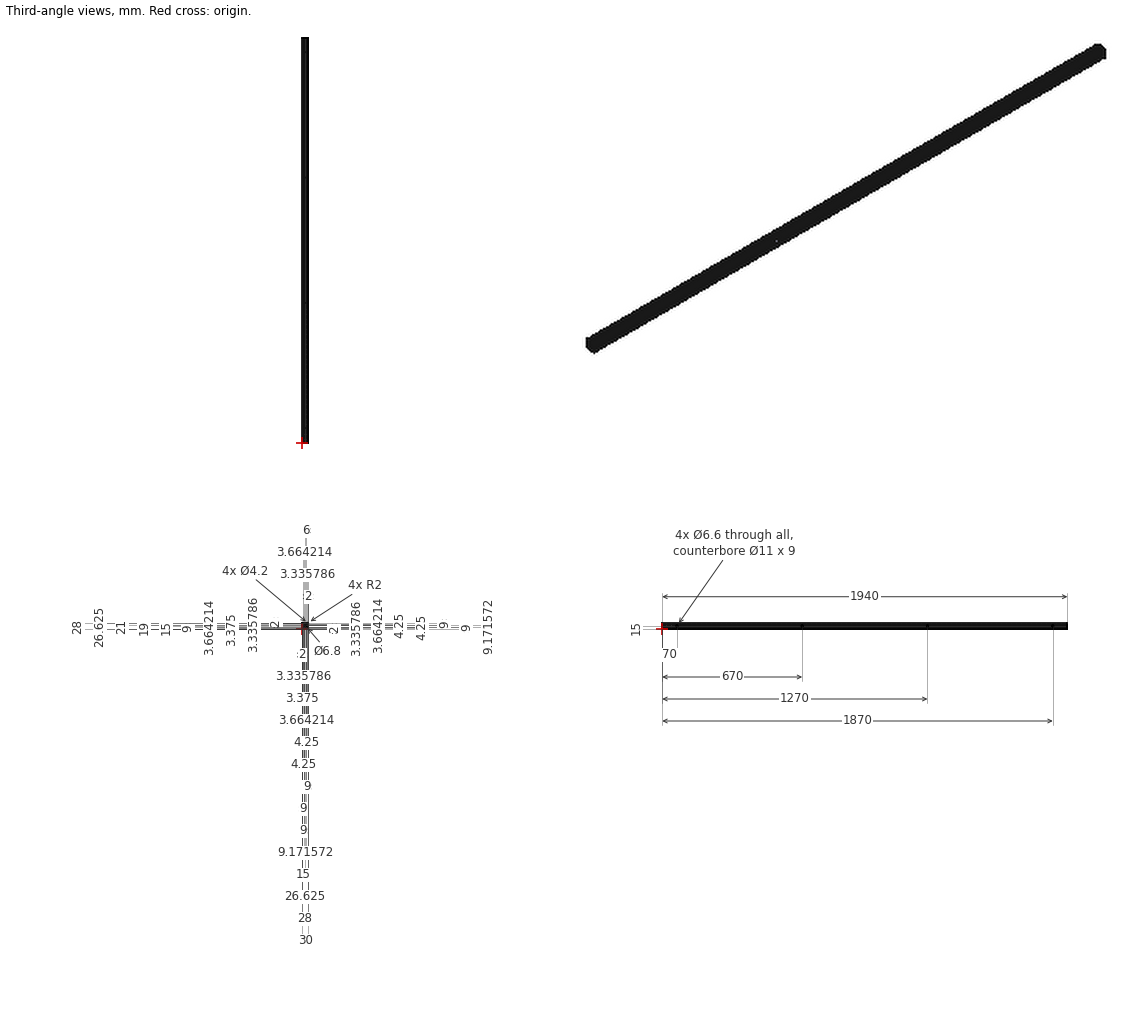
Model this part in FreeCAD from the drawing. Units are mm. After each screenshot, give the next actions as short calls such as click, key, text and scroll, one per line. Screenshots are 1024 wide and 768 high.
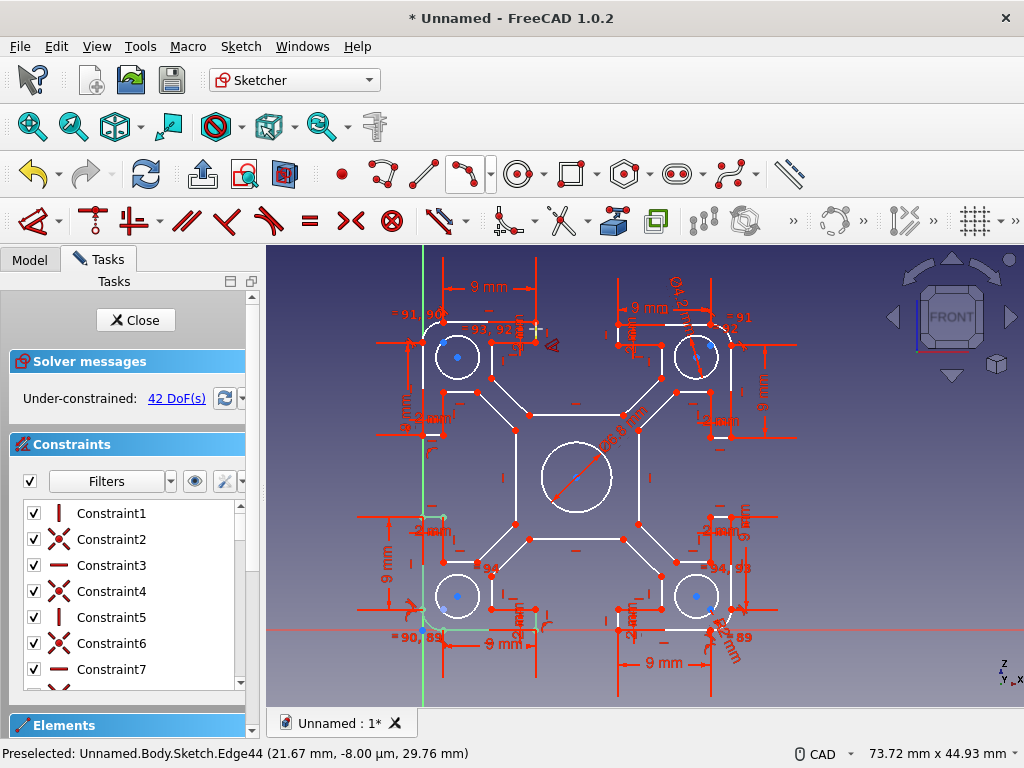
click(624, 539)
click(389, 585)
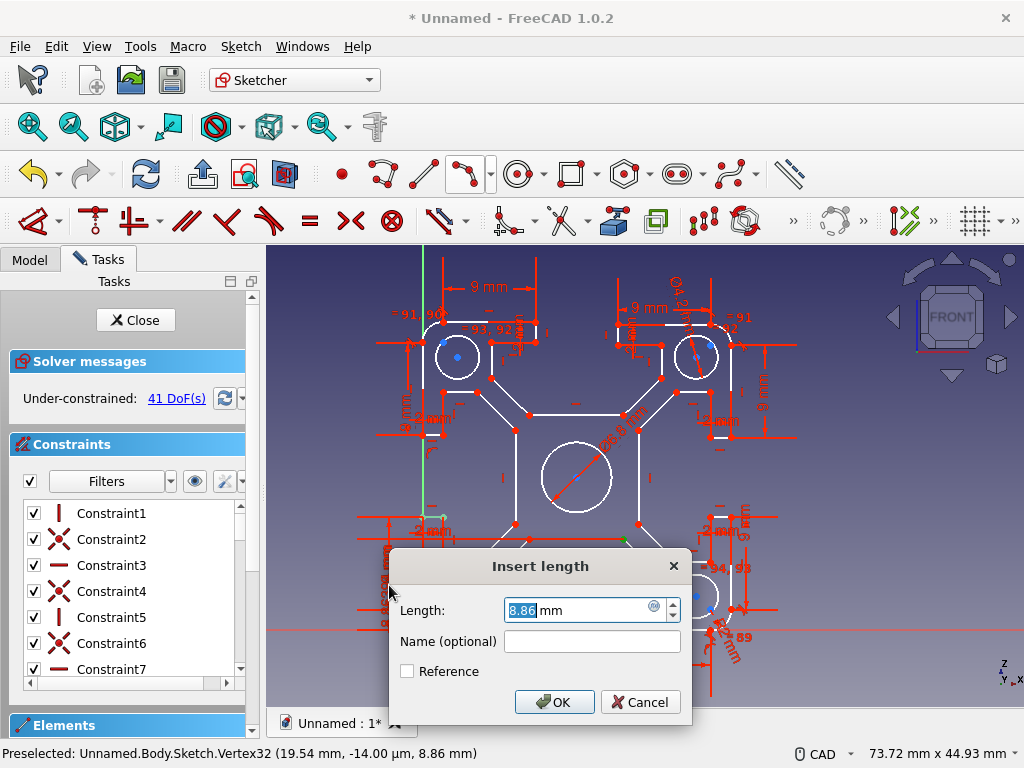
text(9)
key(Return)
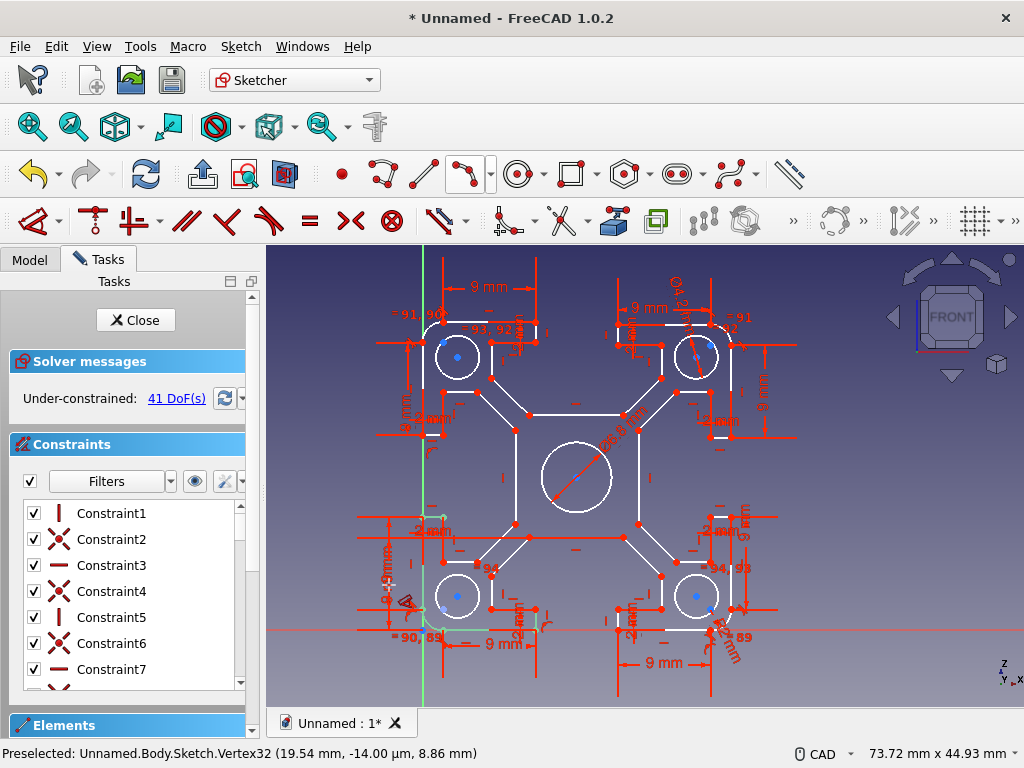
click(516, 524)
click(469, 490)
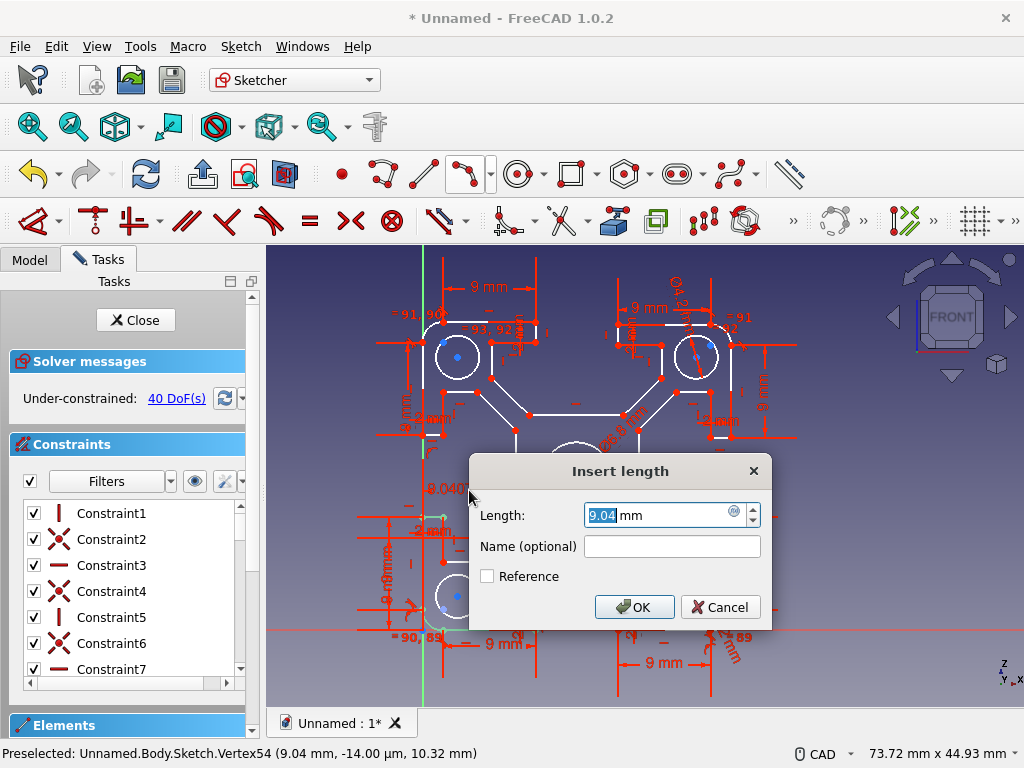
text(9)
key(Return)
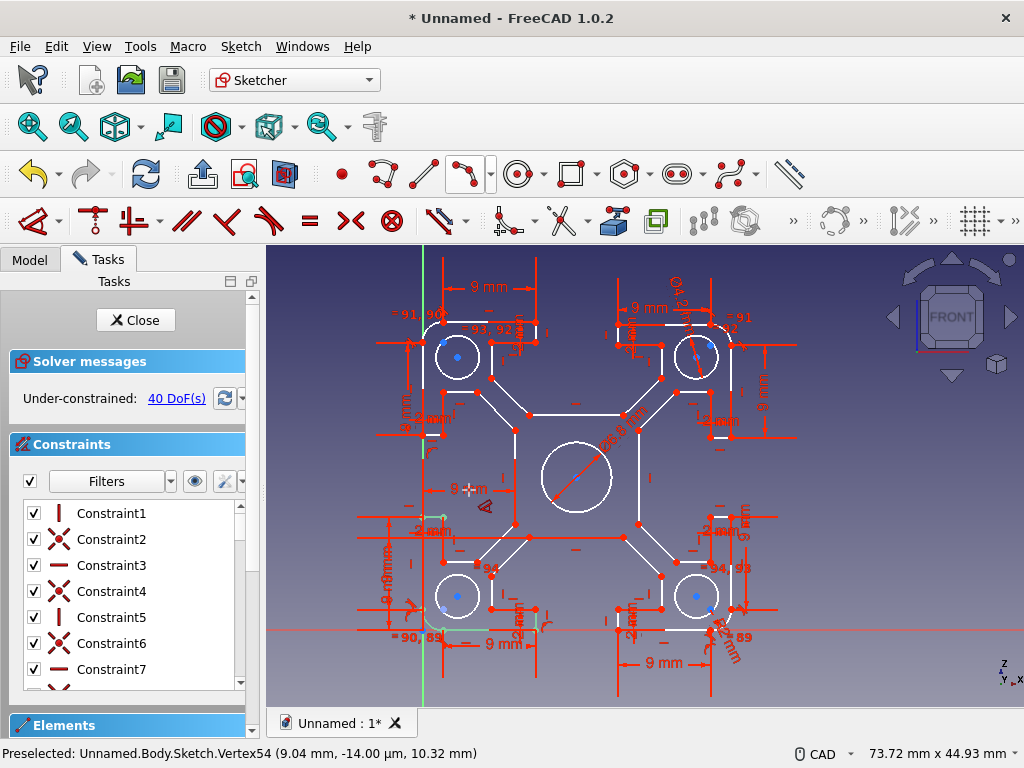
click(577, 477)
click(500, 443)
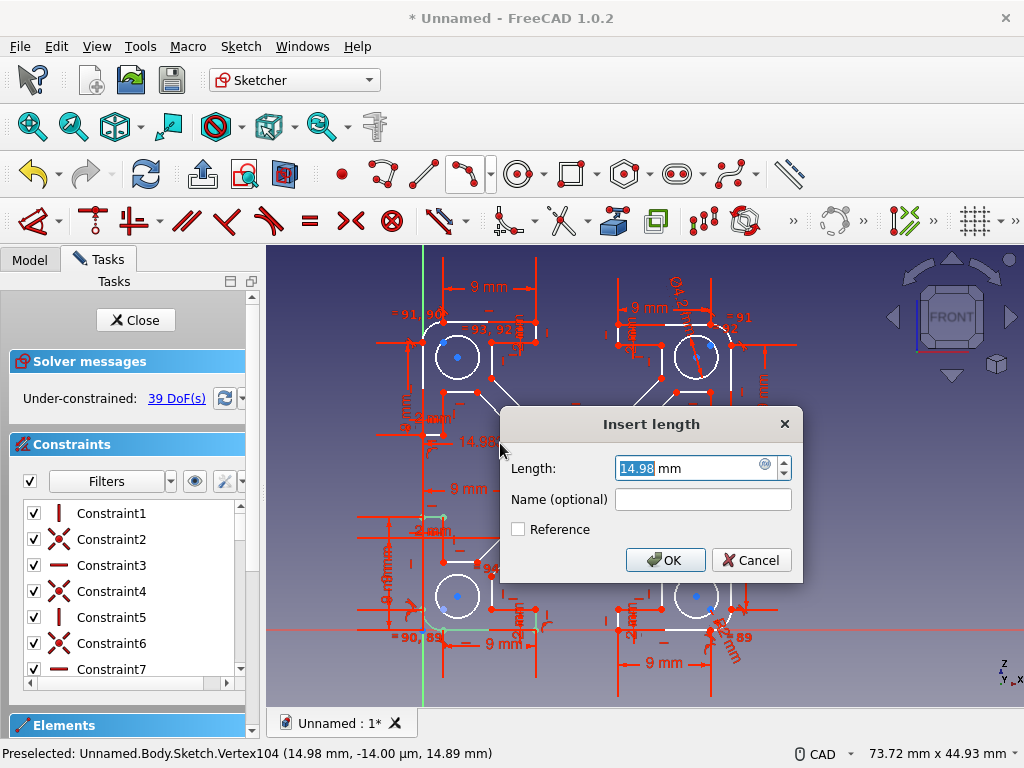
text(15)
key(Return)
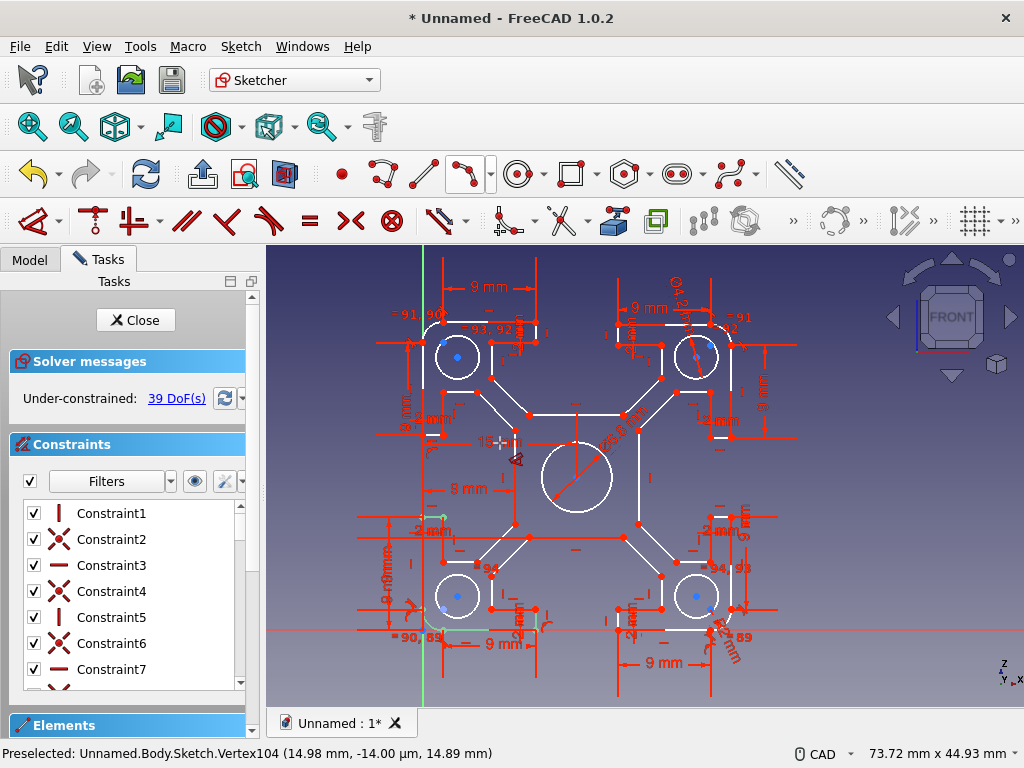
click(577, 477)
click(389, 500)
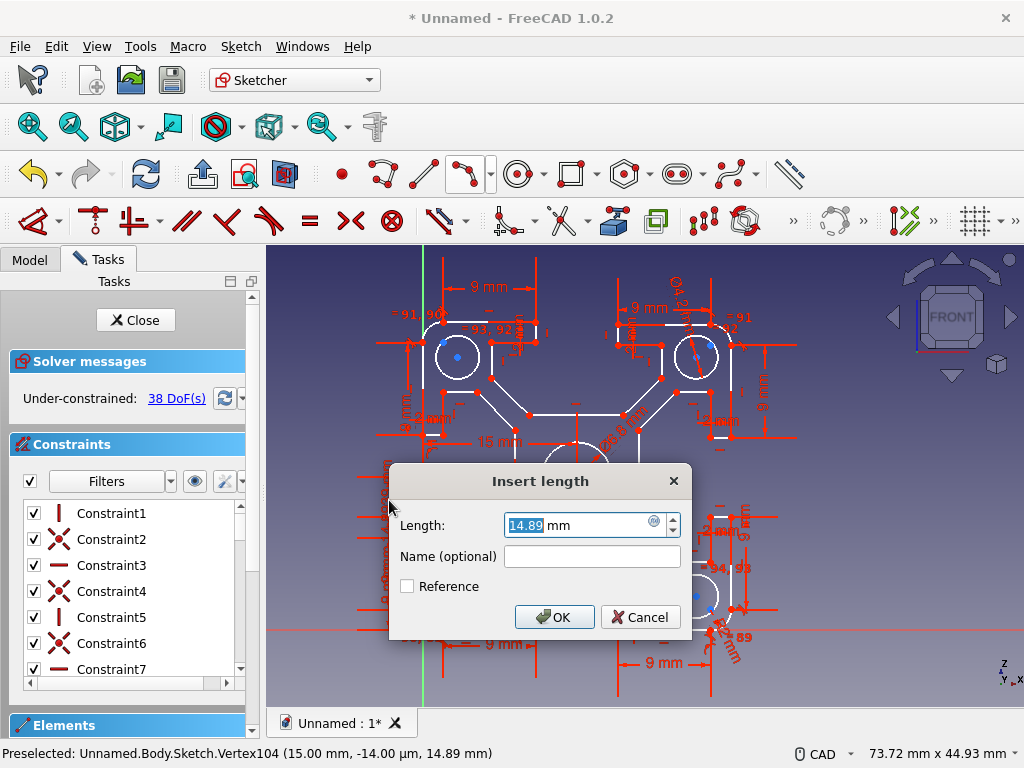
text(15)
key(Return)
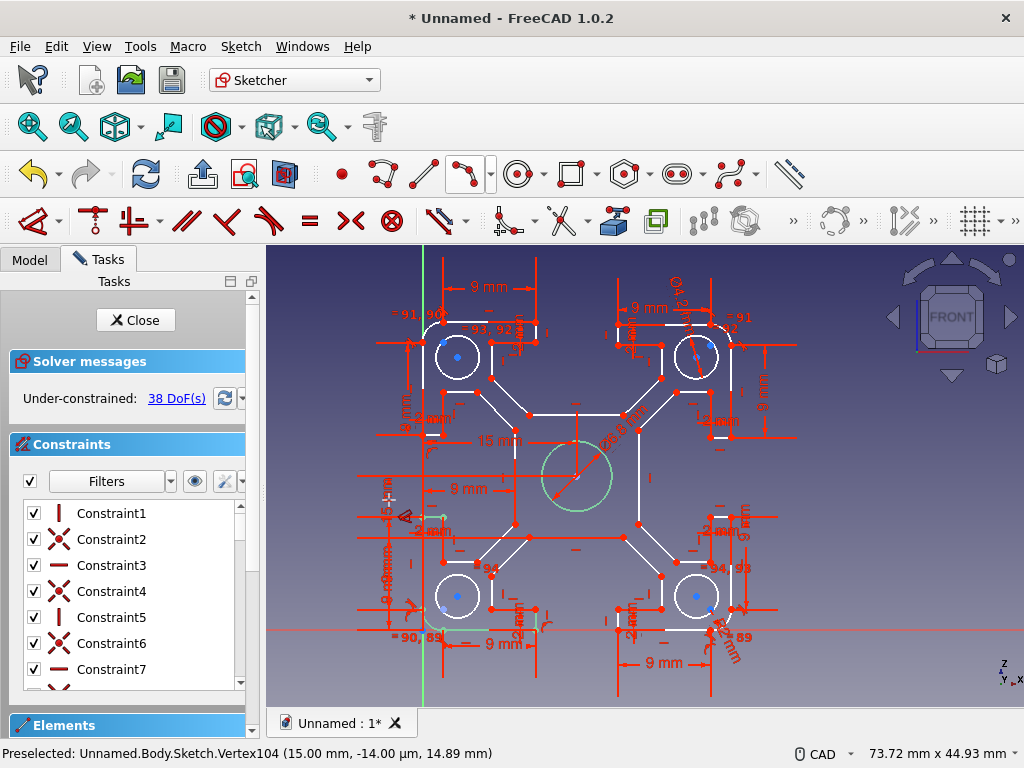
click(639, 430)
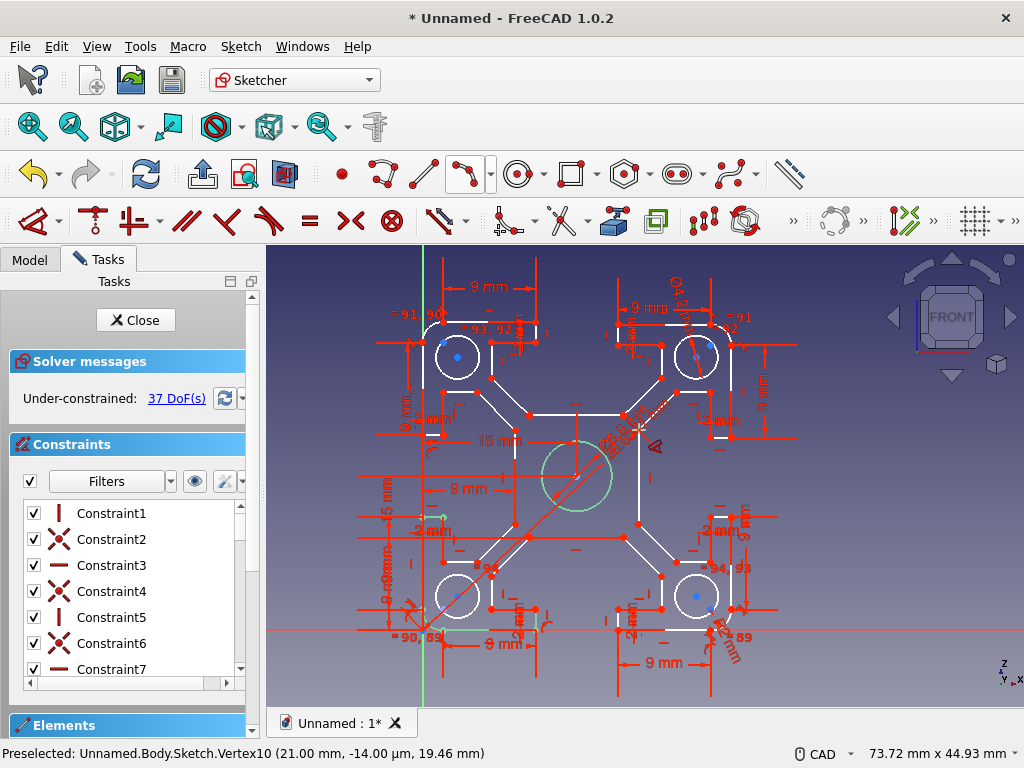
click(577, 476)
click(608, 396)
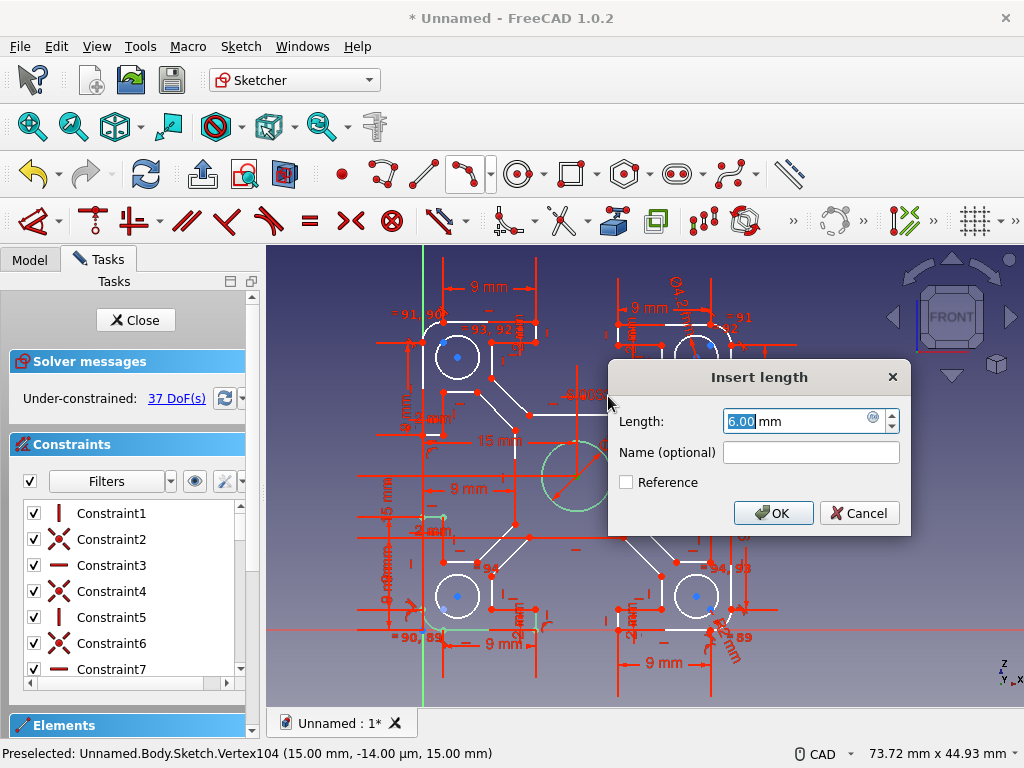
text(6)
key(Return)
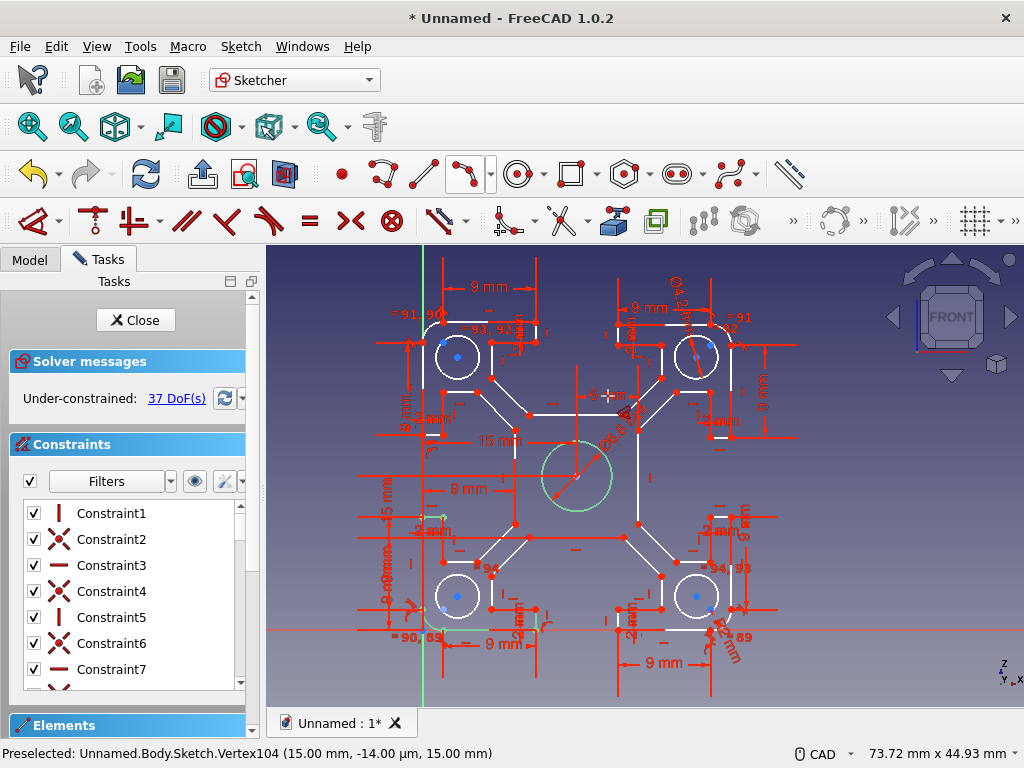
click(731, 345)
click(577, 664)